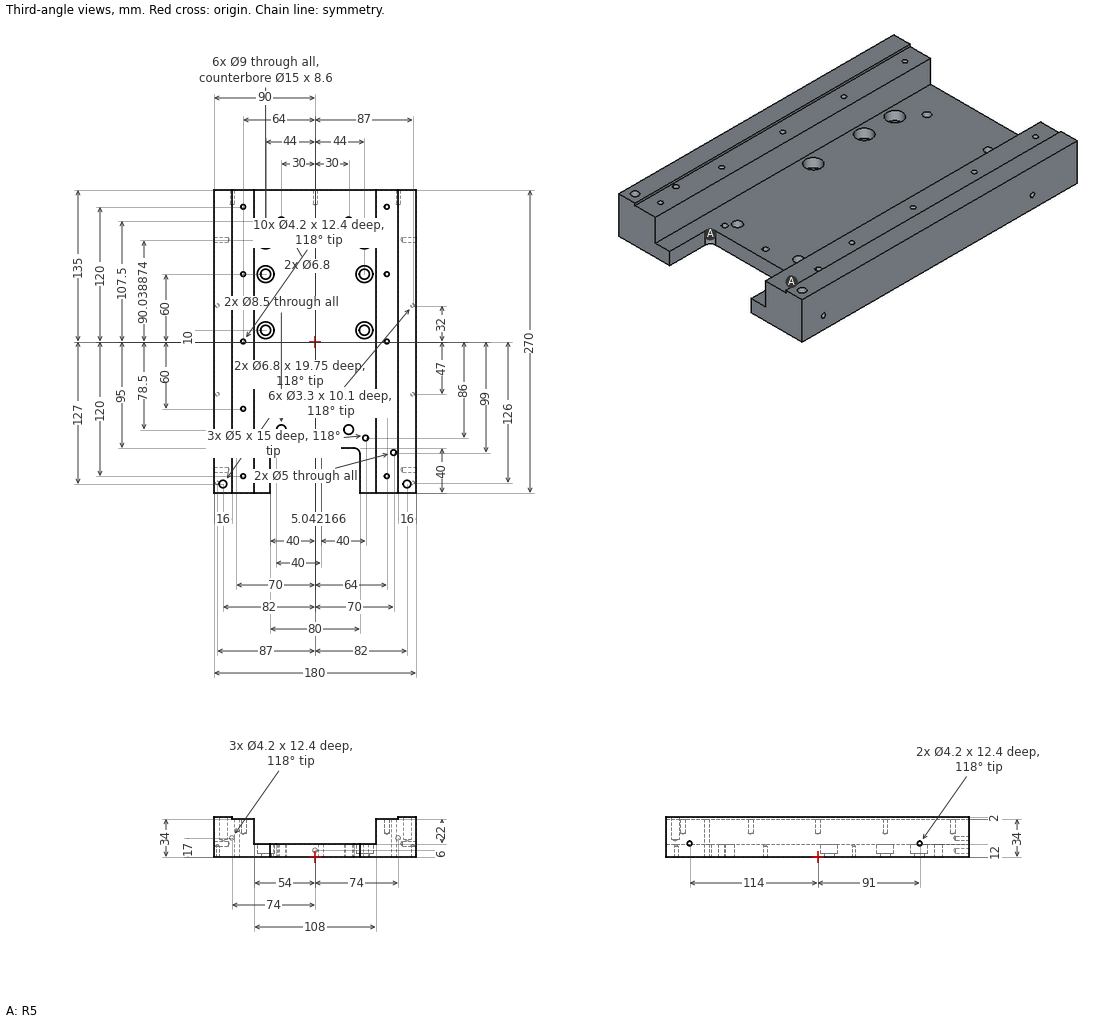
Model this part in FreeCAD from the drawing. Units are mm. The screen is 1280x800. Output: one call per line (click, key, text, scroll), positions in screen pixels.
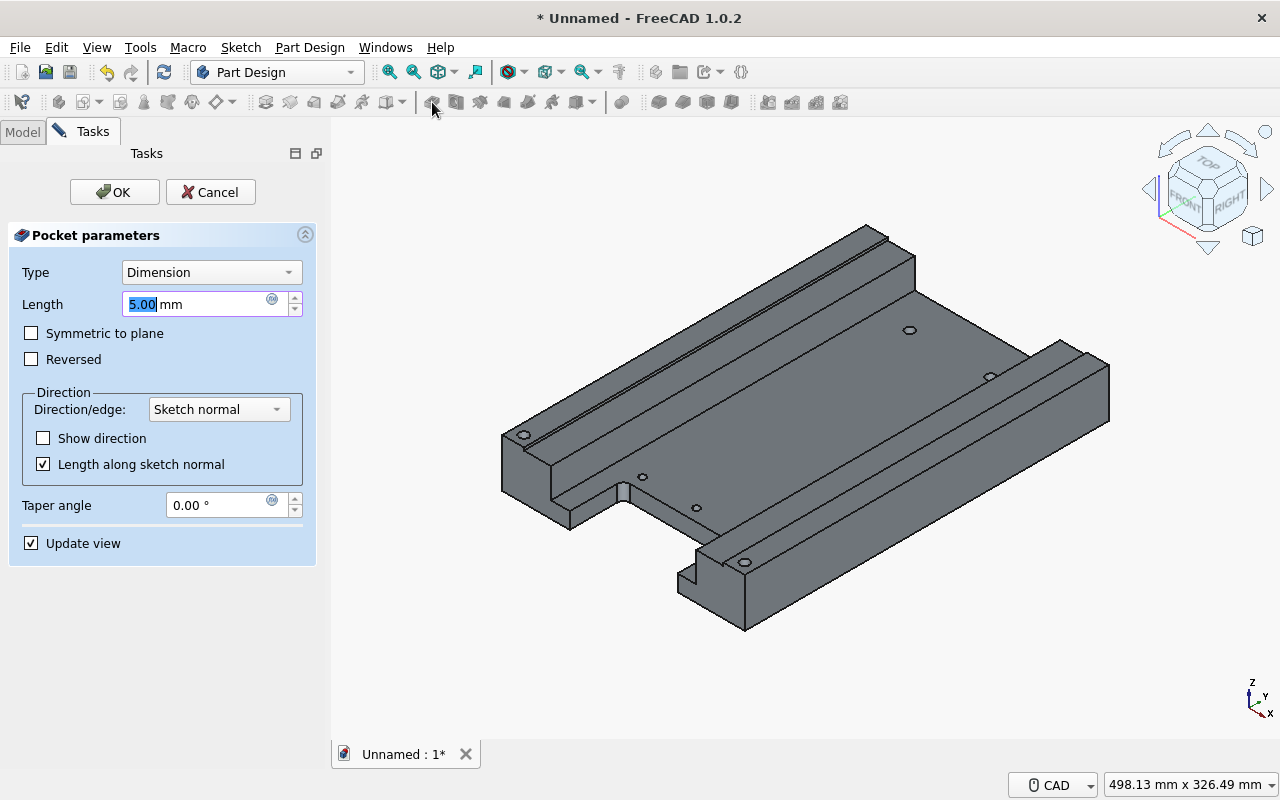
click(212, 272)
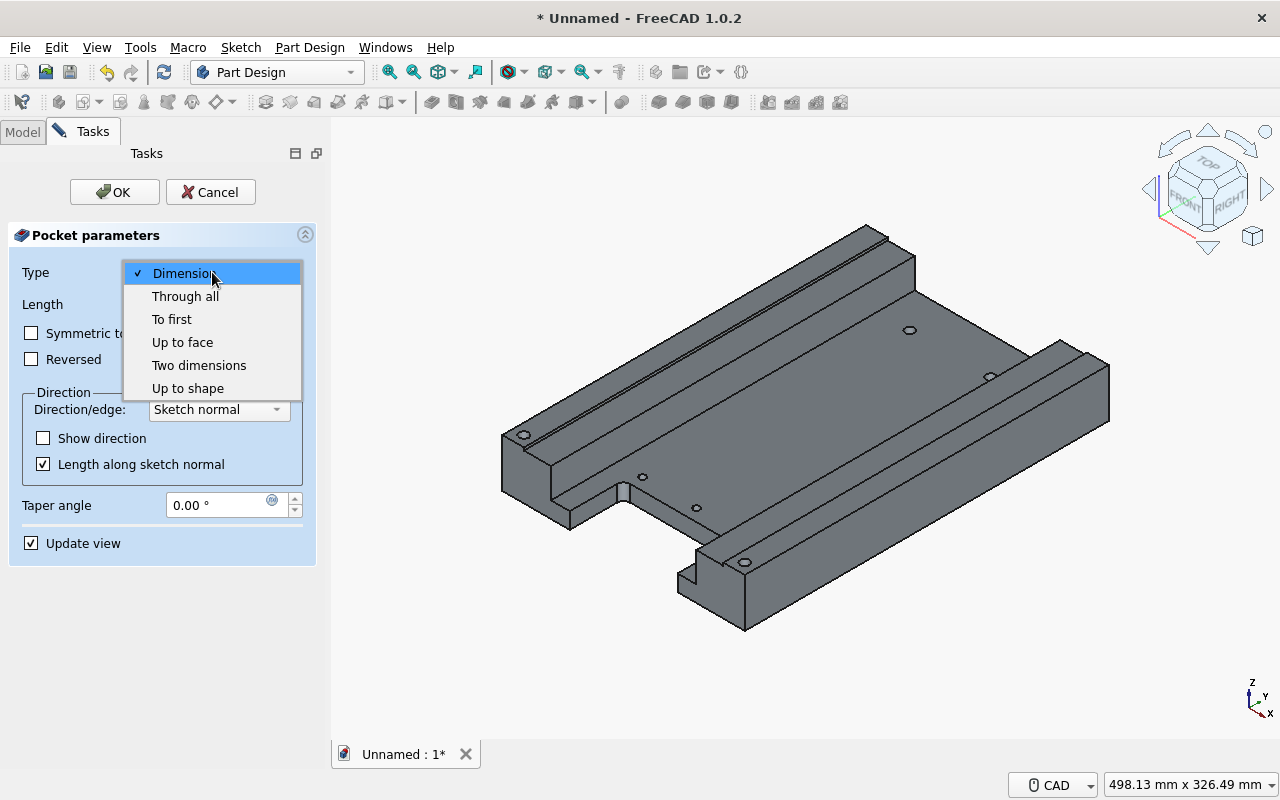
click(212, 296)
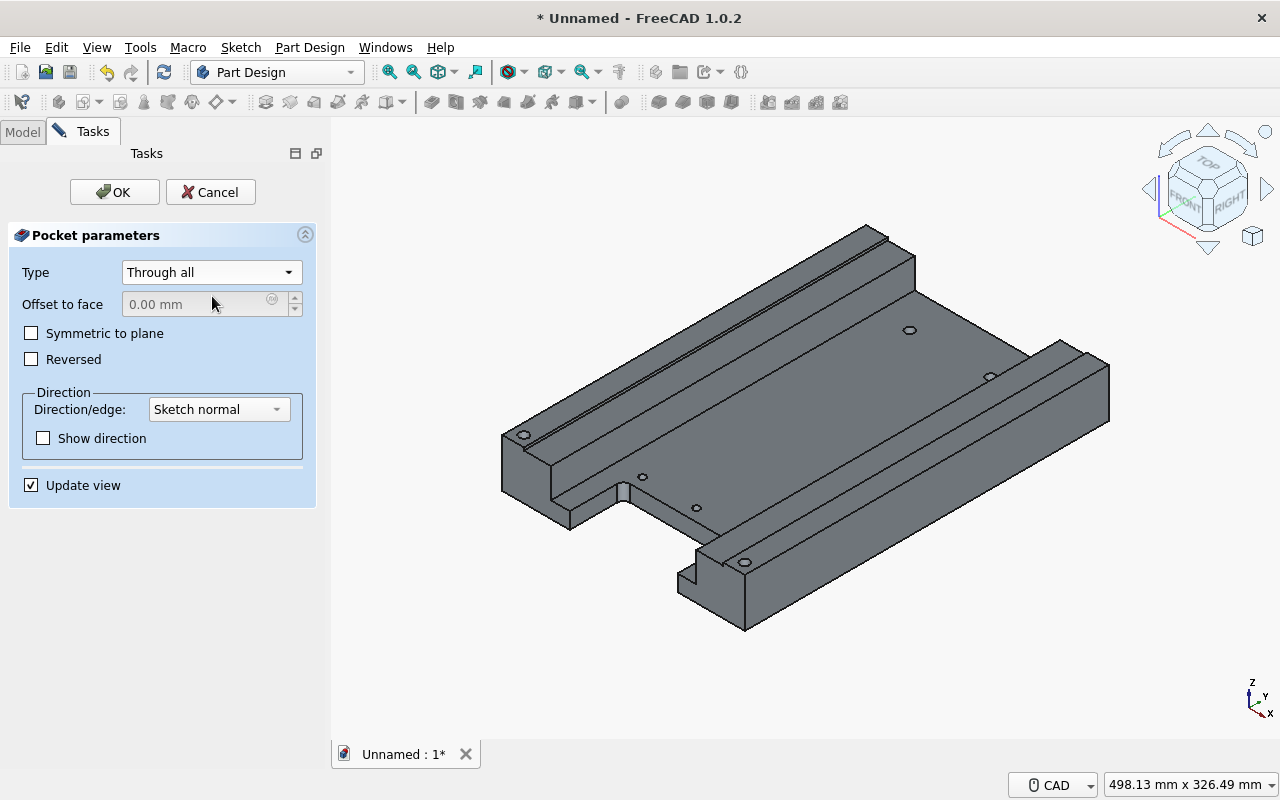
click(115, 192)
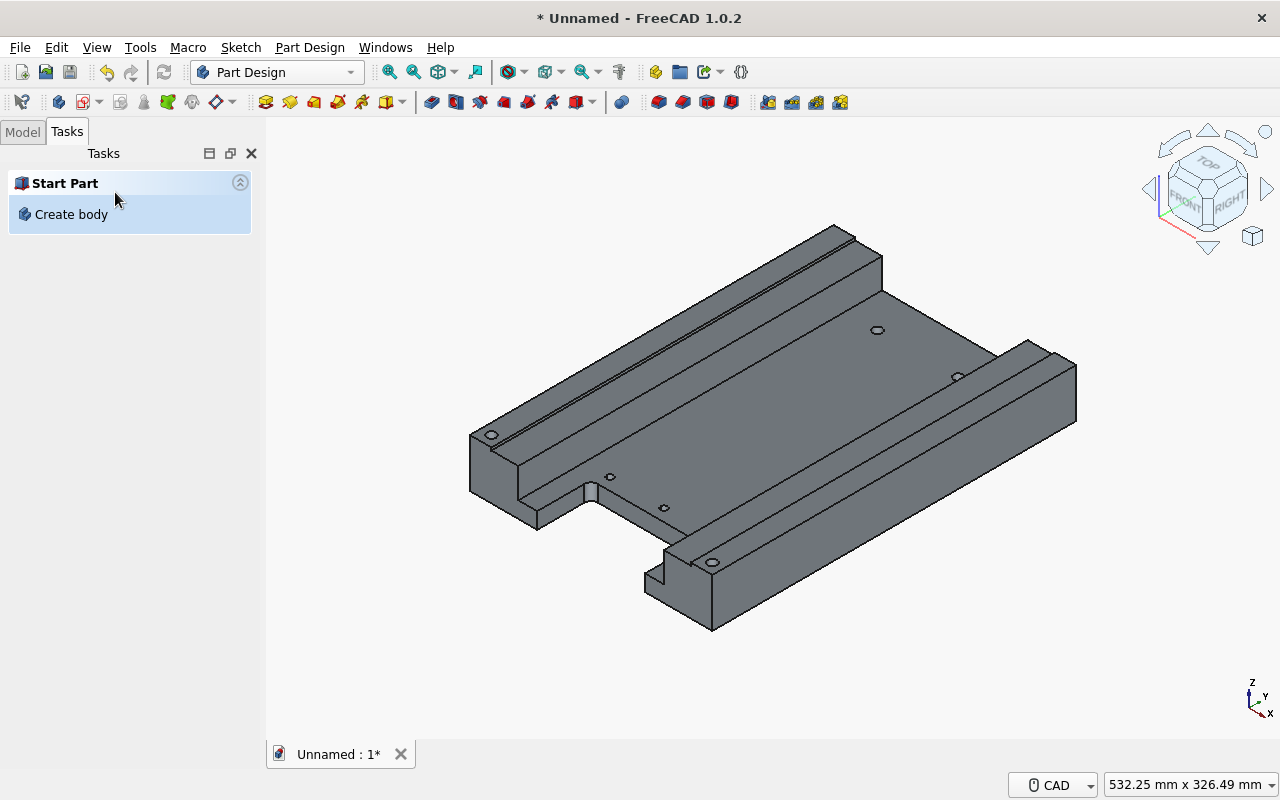
click(825, 406)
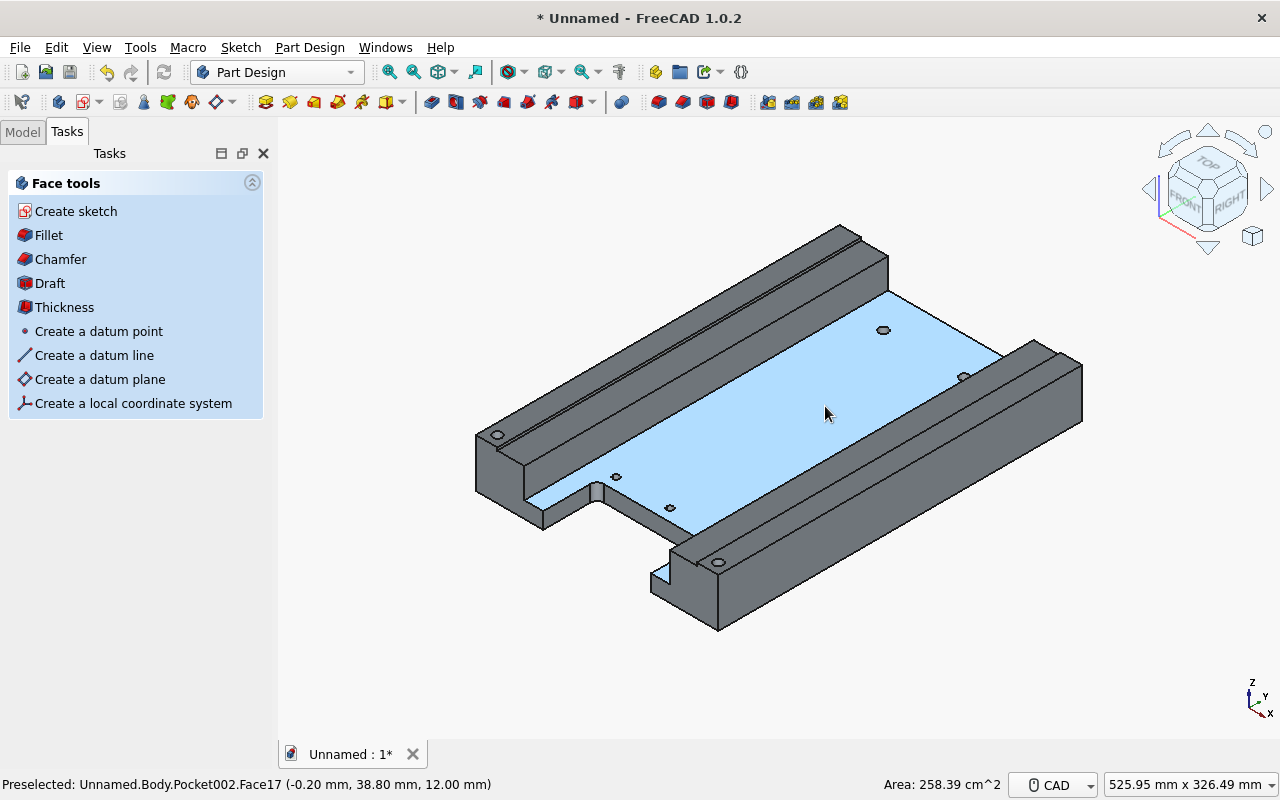
click(84, 102)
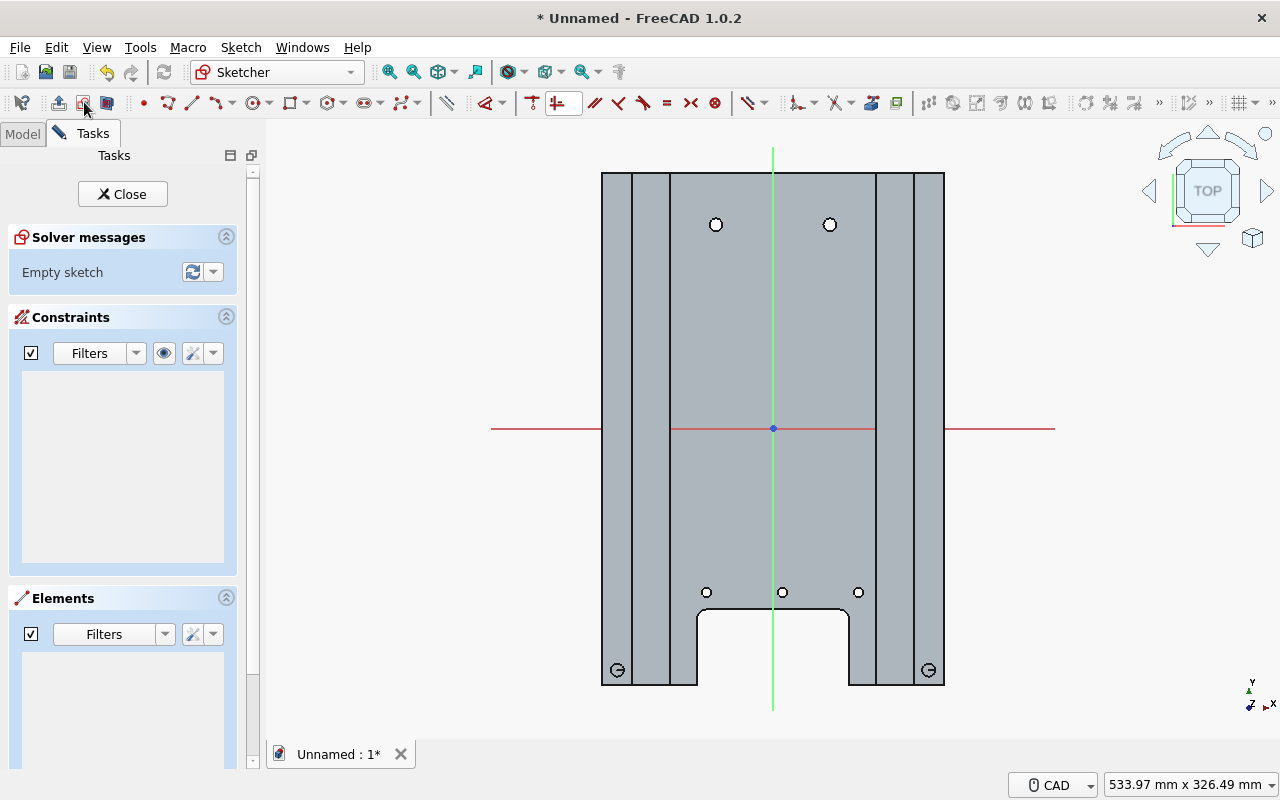
scroll(813, 553, up, 5)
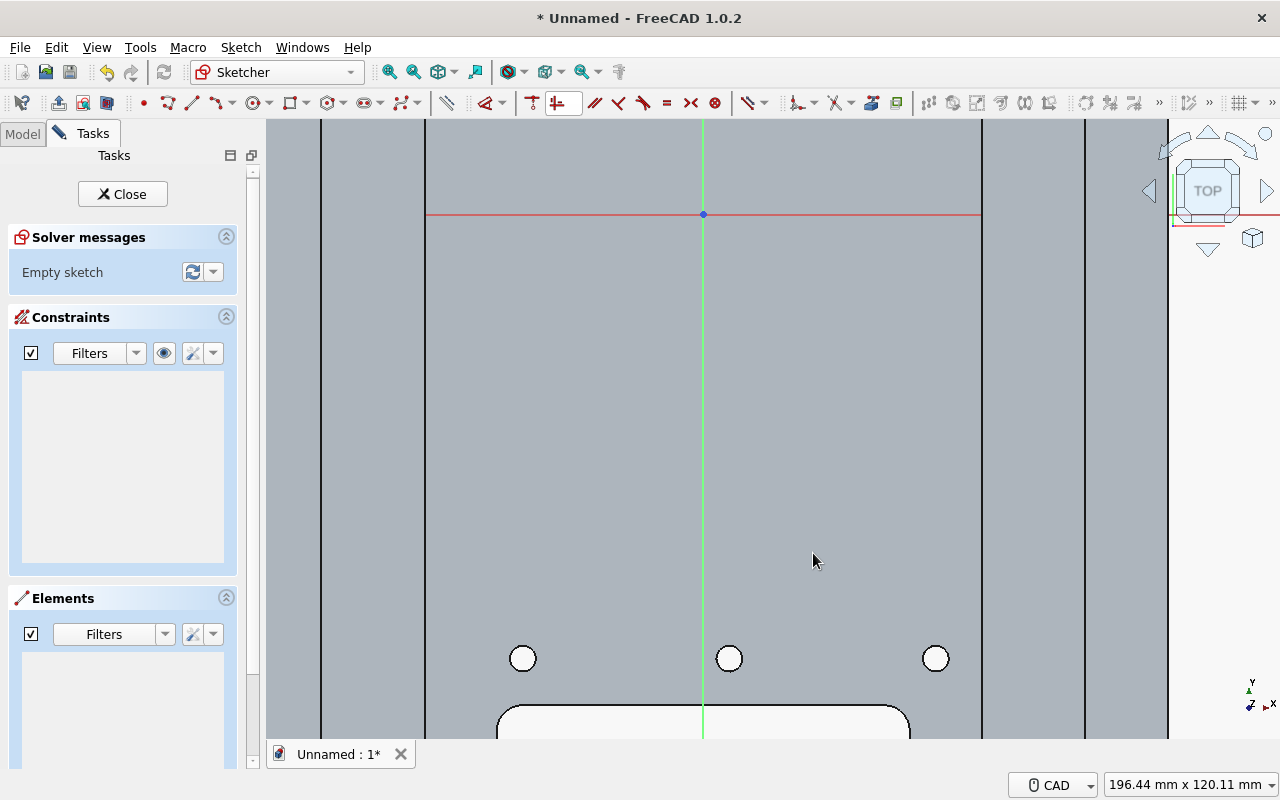
key(g)
key(c)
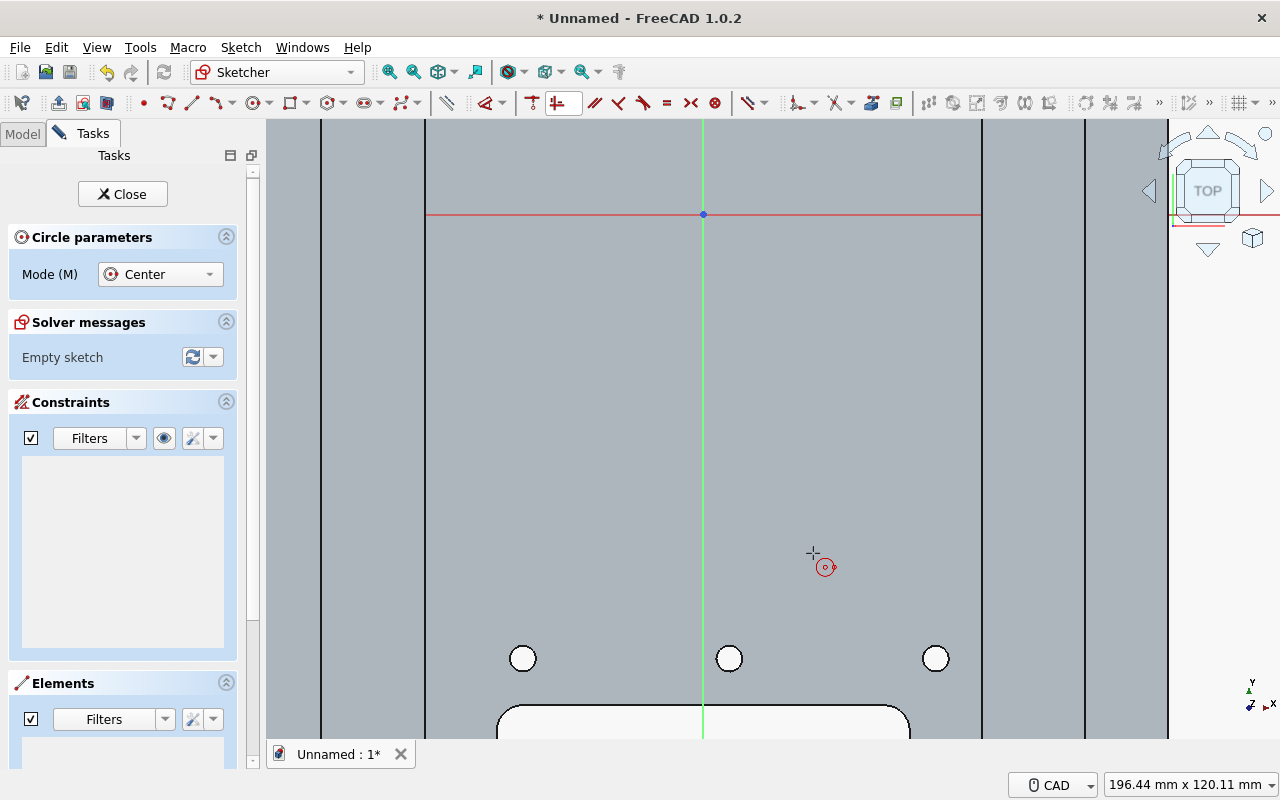
click(548, 620)
move(564, 604)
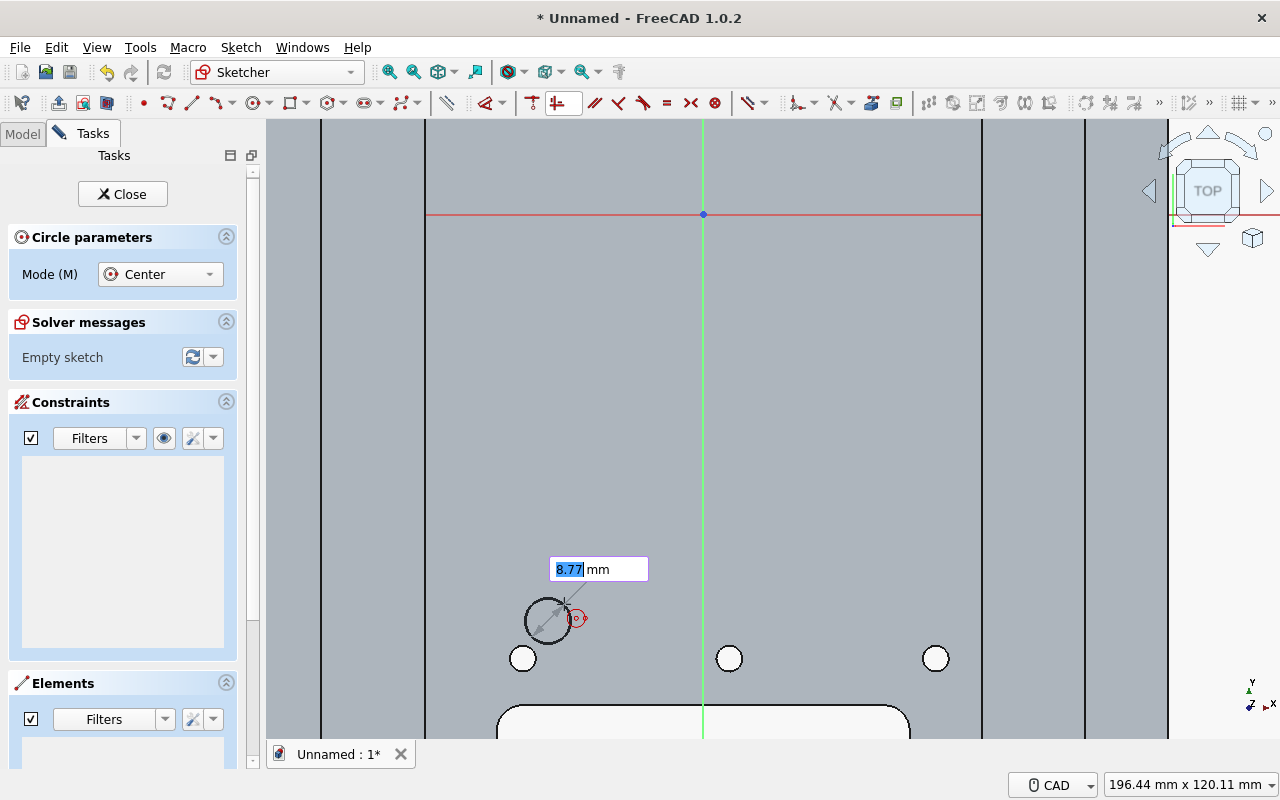
text(8.5)
key(Return)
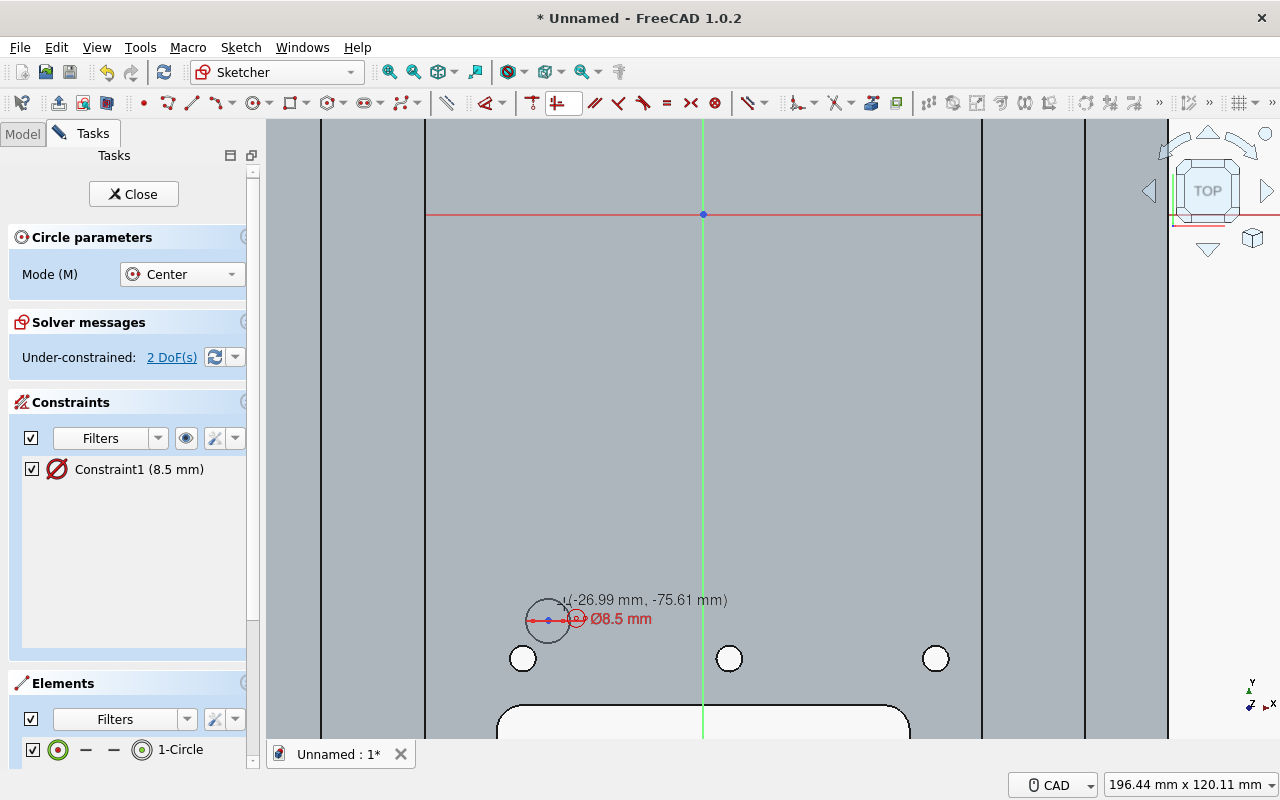
click(858, 620)
move(874, 604)